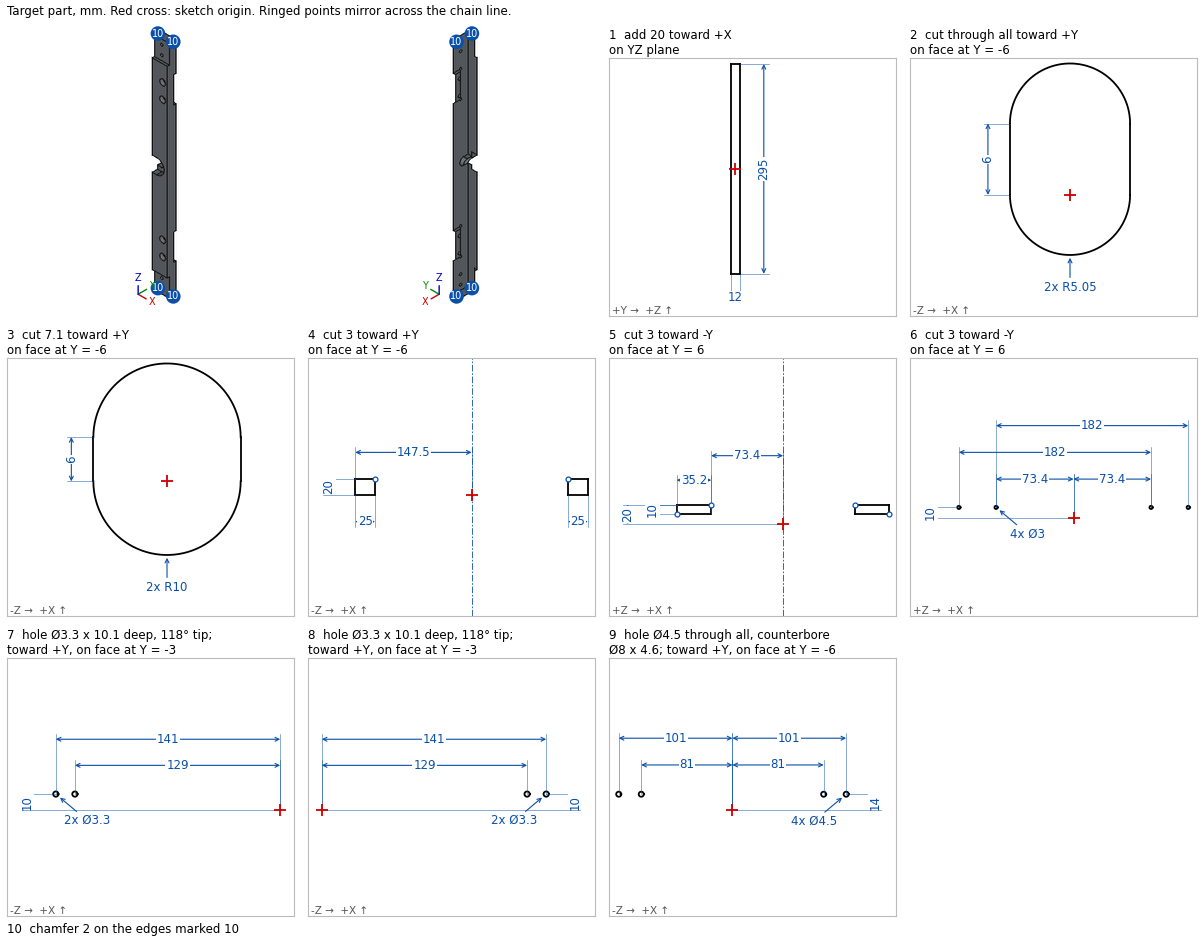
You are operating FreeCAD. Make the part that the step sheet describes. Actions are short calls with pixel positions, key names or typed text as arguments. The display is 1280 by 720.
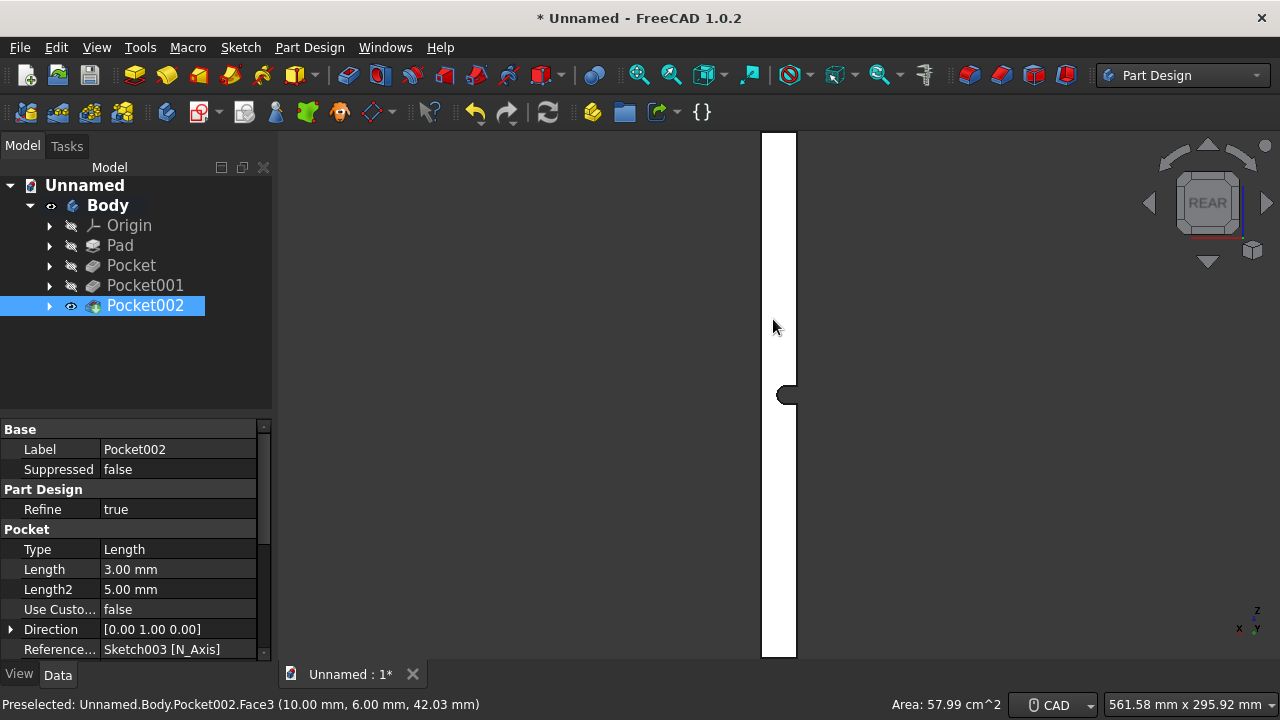
click(200, 112)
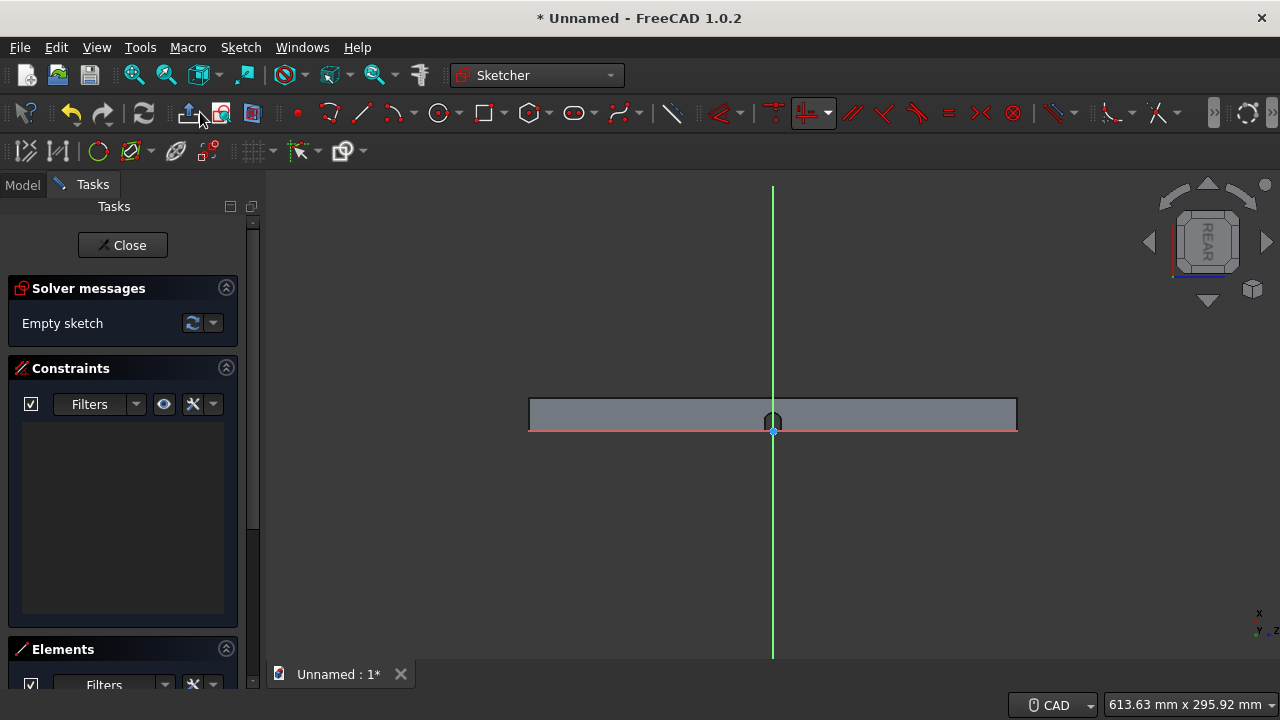
scroll(912, 414, up, 2)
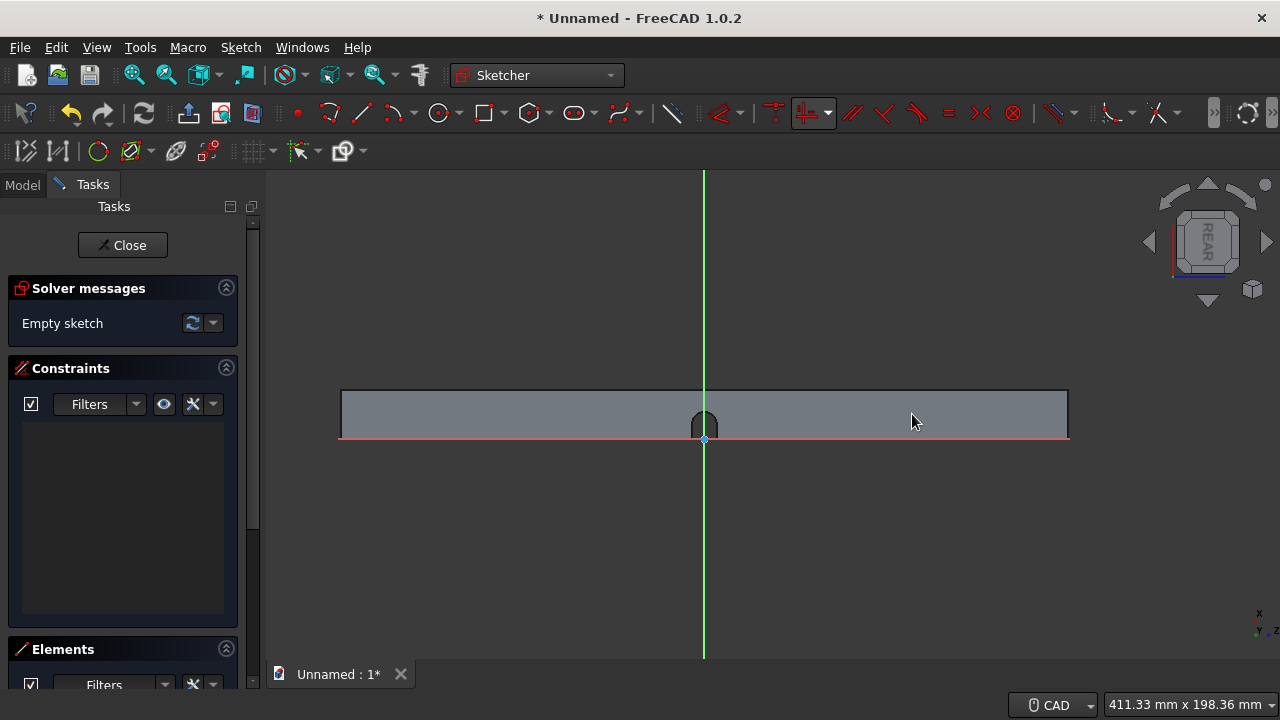
click(484, 114)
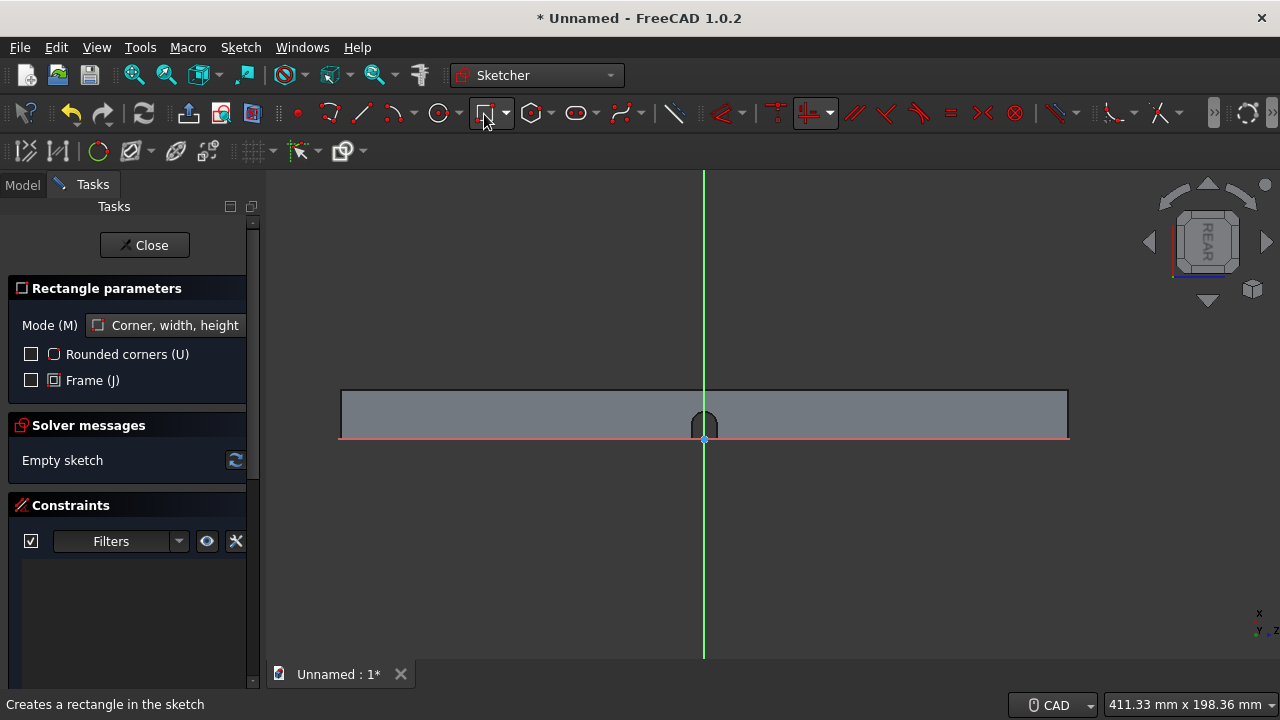
click(437, 390)
click(523, 414)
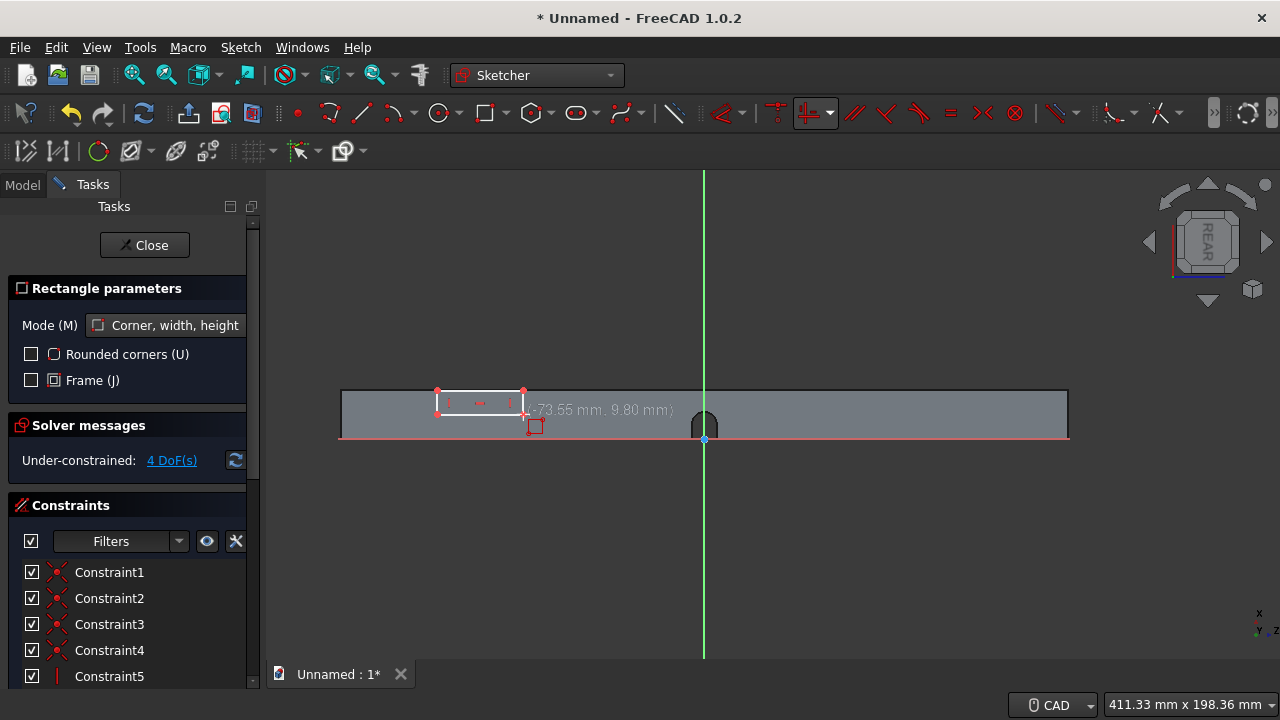
click(885, 390)
click(972, 414)
key(Escape)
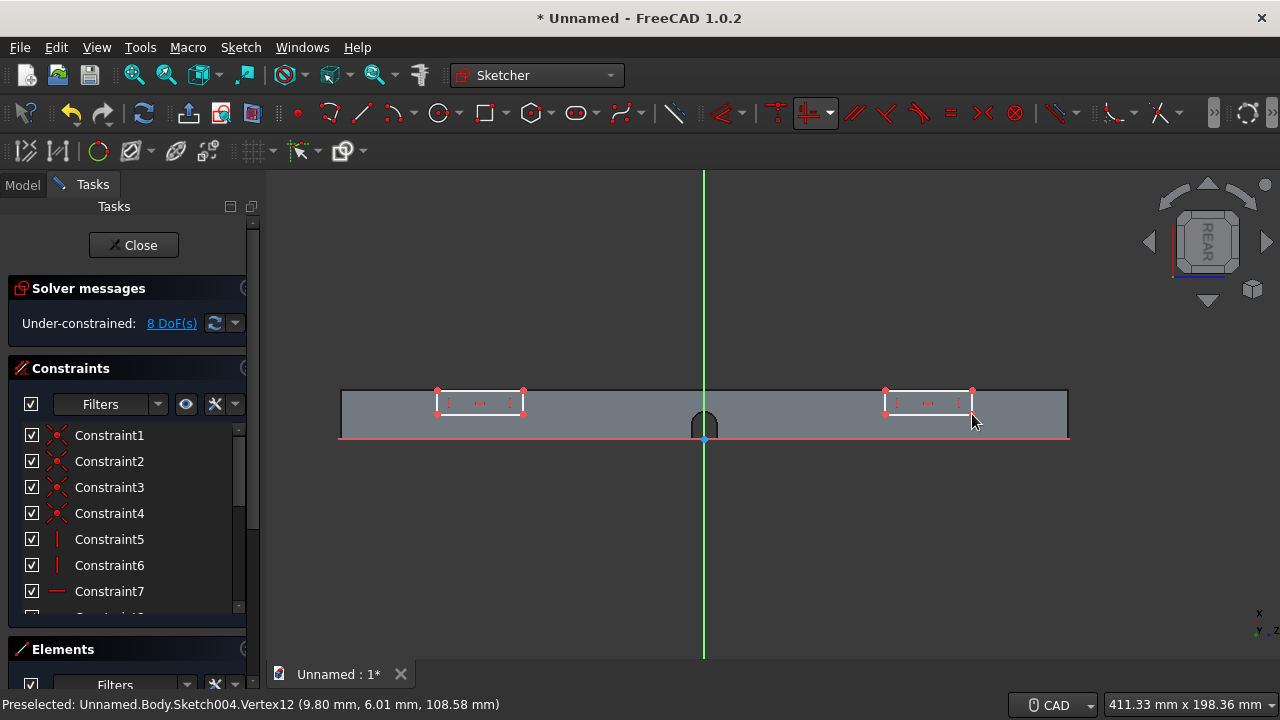
click(523, 391)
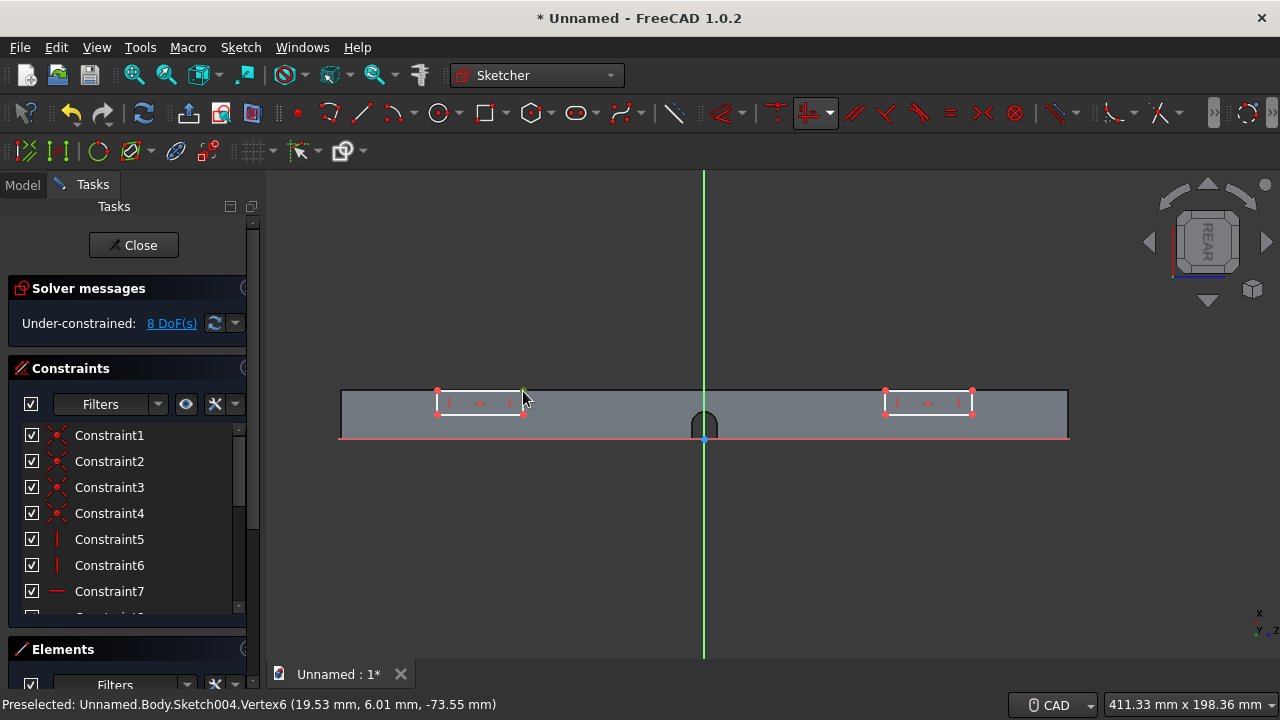
click(885, 391)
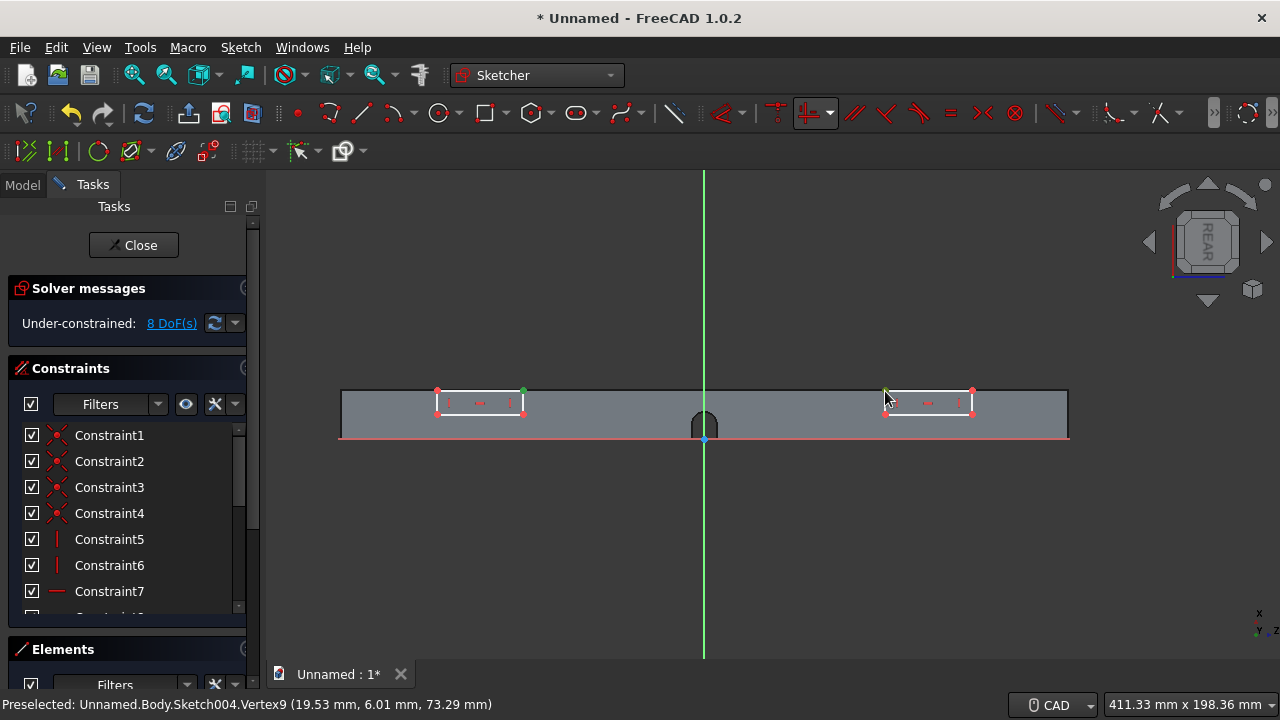
click(704, 600)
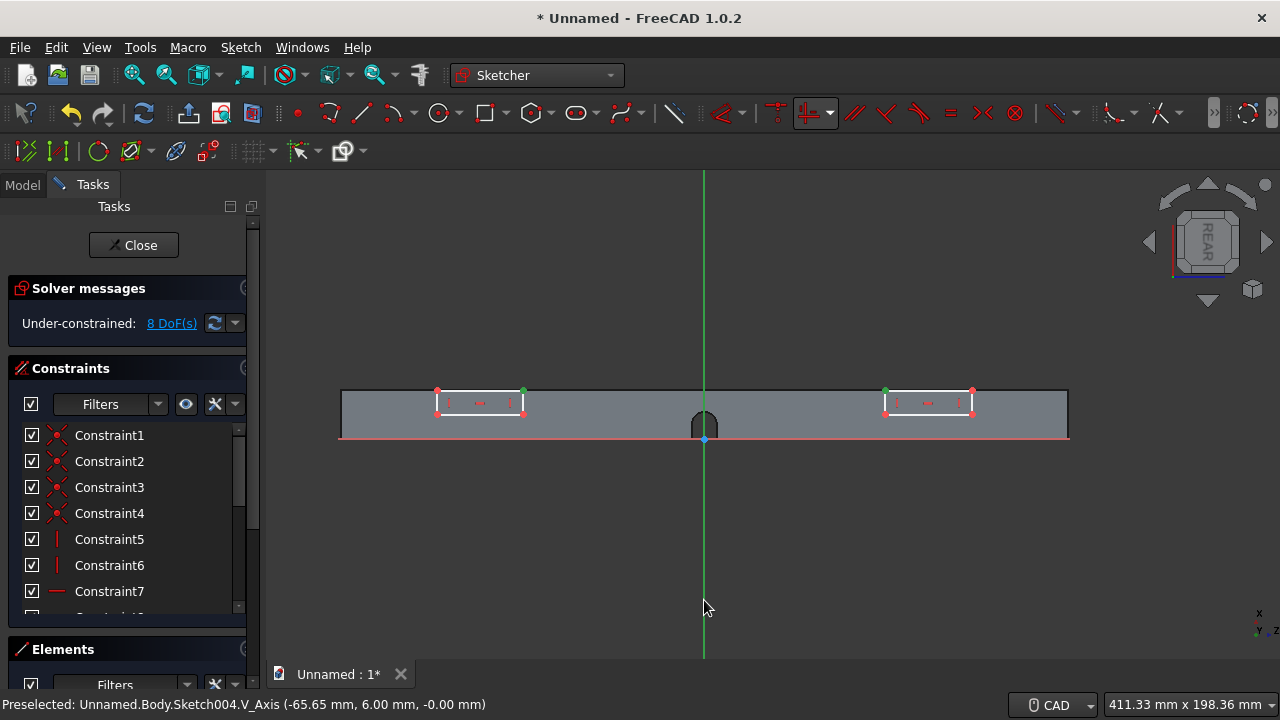
click(984, 114)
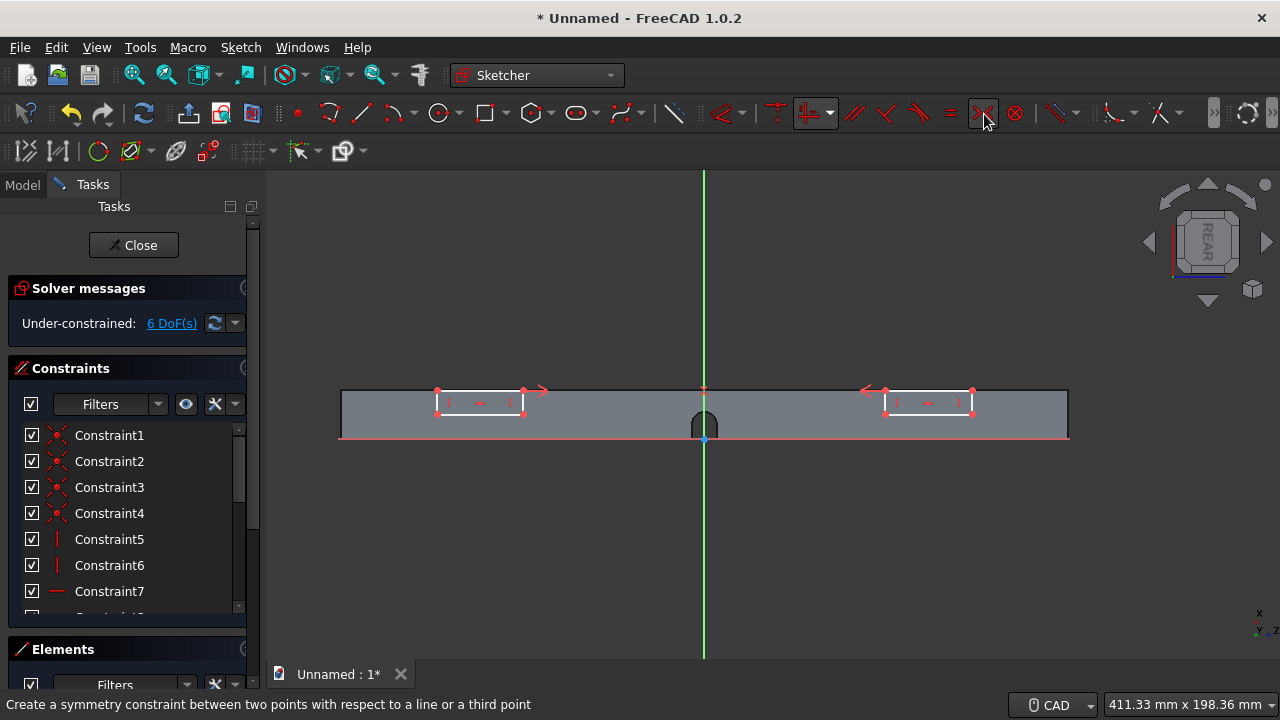
click(437, 415)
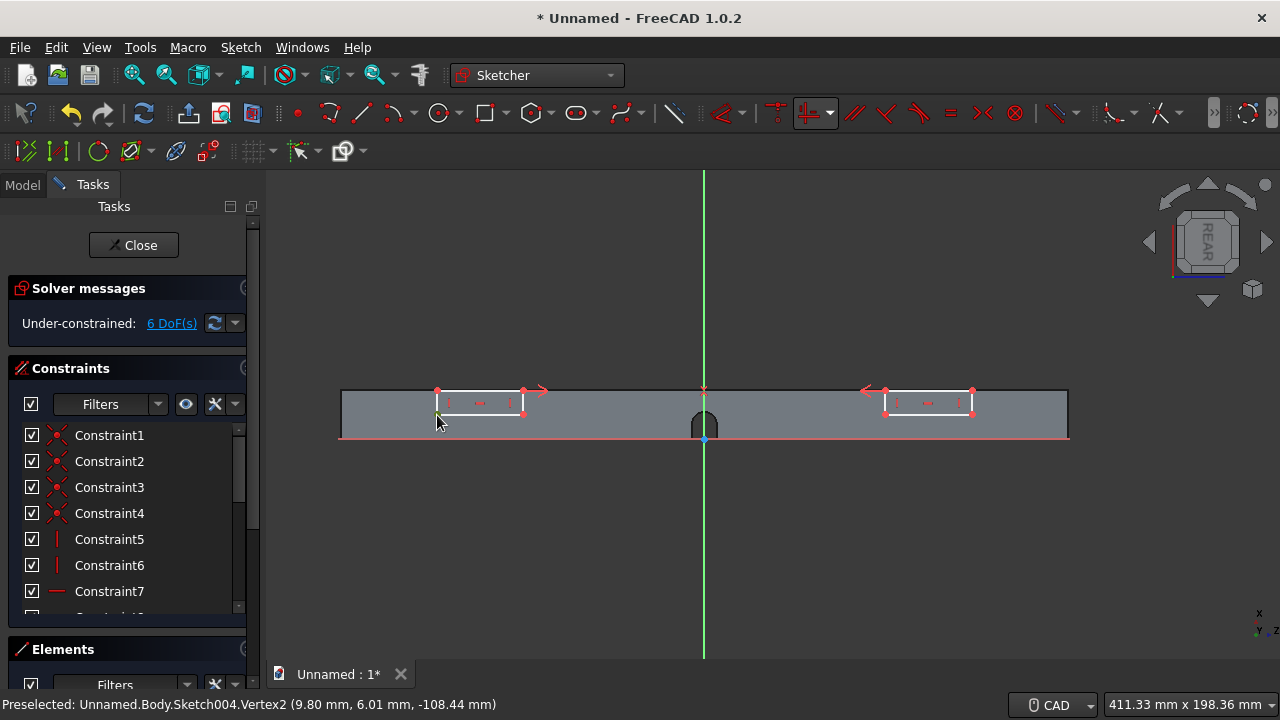
click(972, 415)